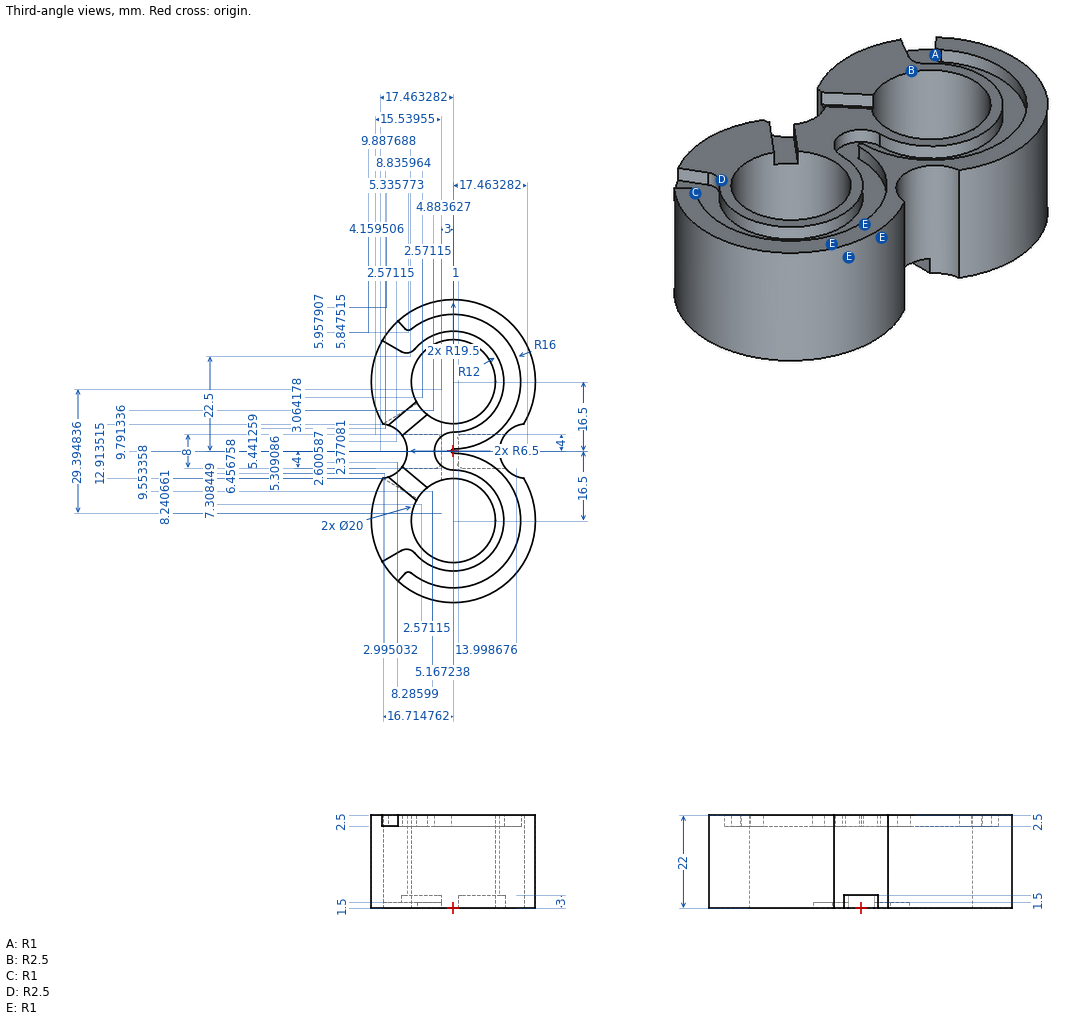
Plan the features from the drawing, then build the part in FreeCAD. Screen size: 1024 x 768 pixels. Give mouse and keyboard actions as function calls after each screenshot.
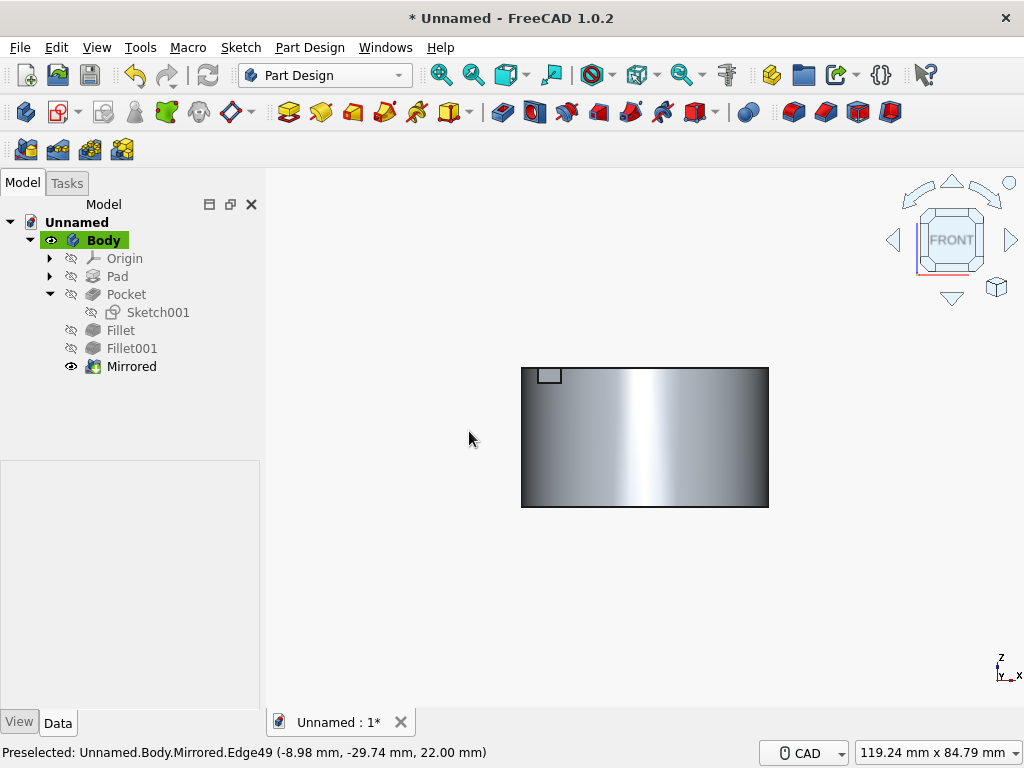
scroll(576, 375, up, 5)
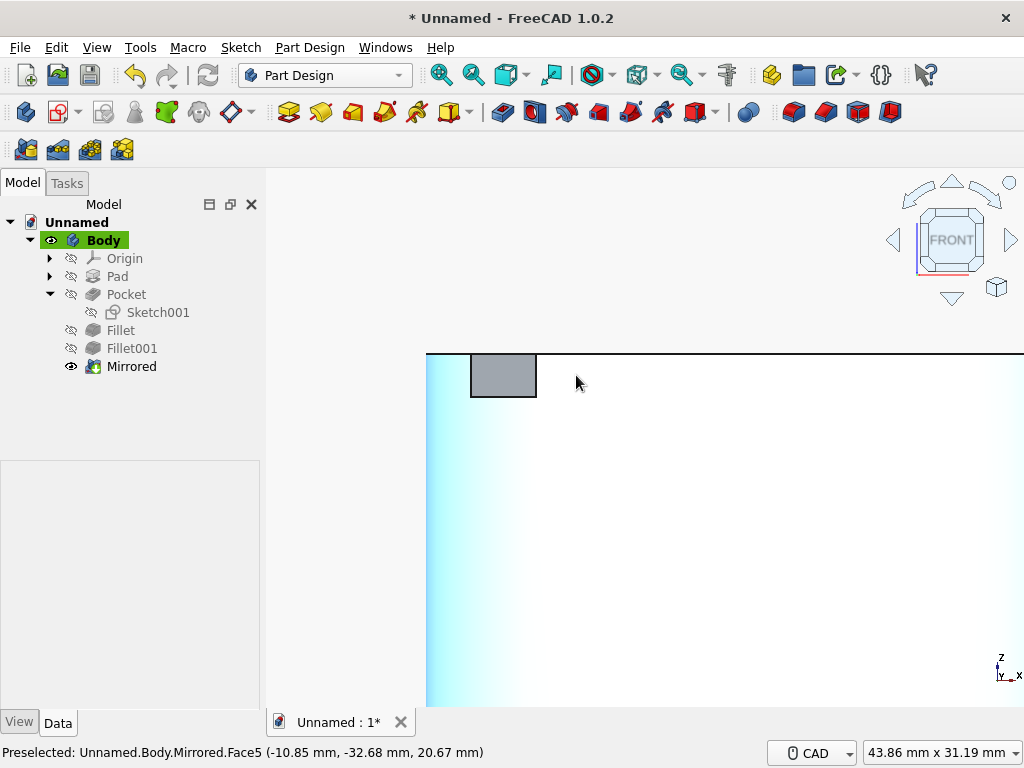
key(v)
key(f)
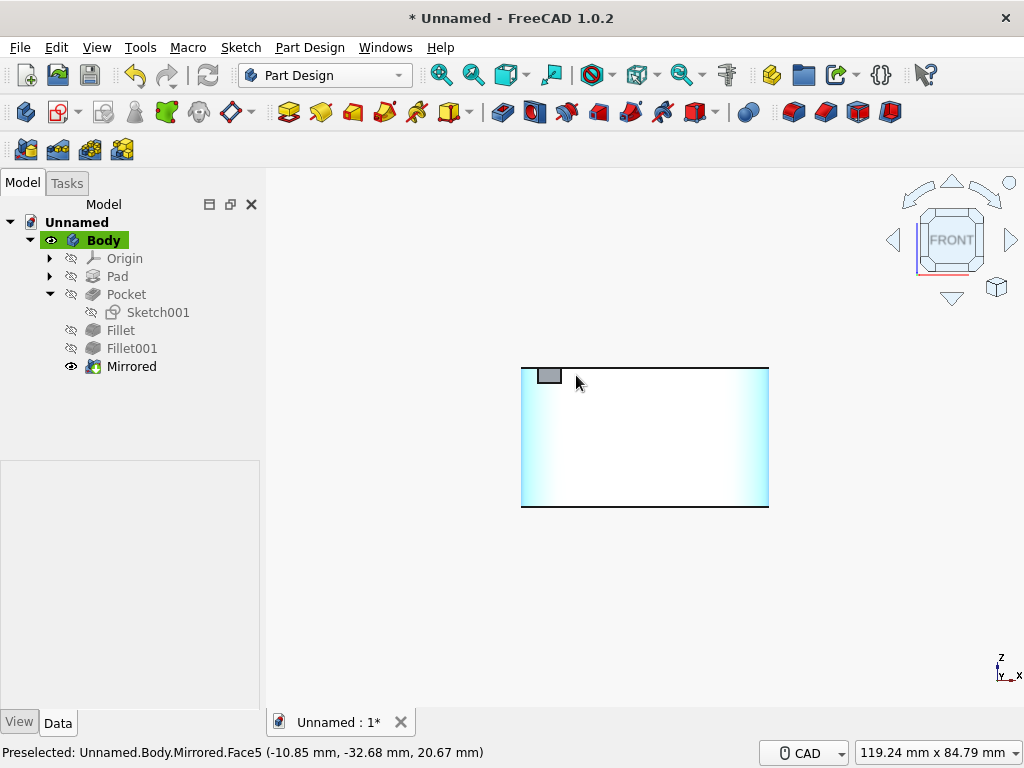
key(3)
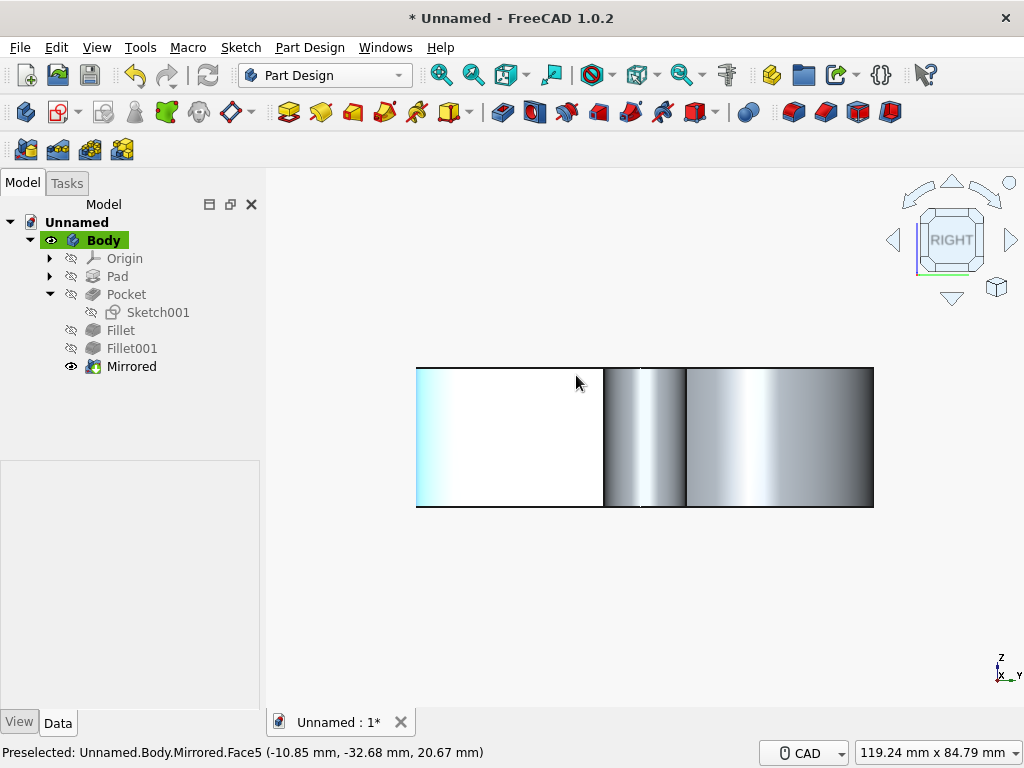
scroll(465, 375, up, 5)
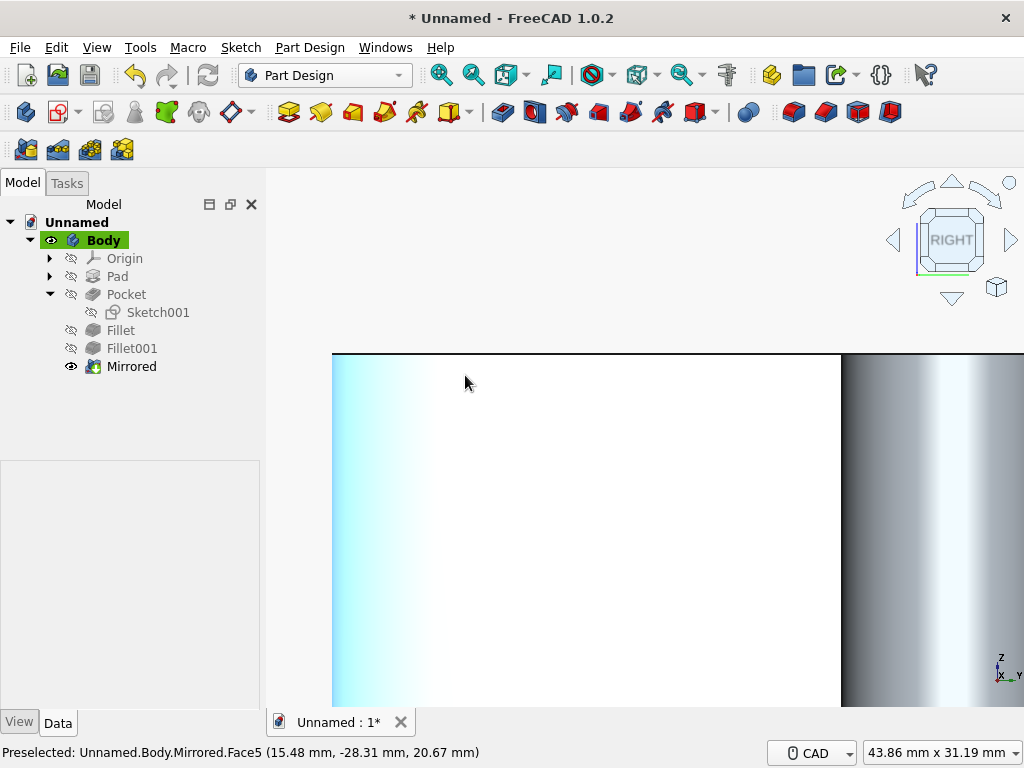
key(v)
key(f)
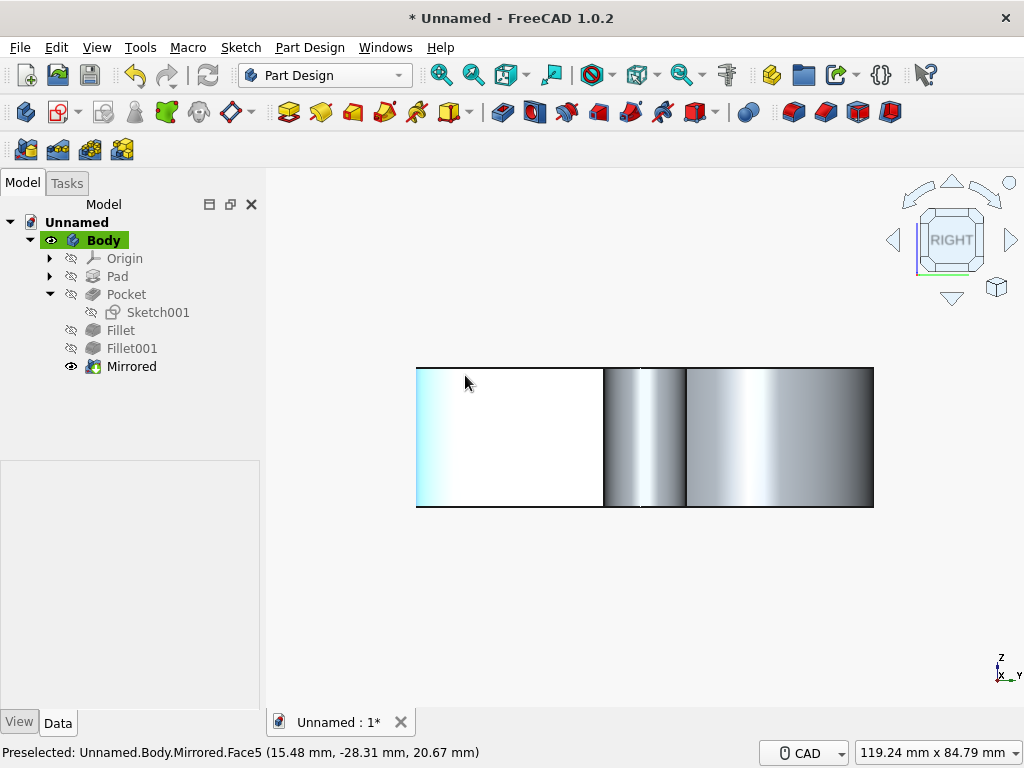
key(5)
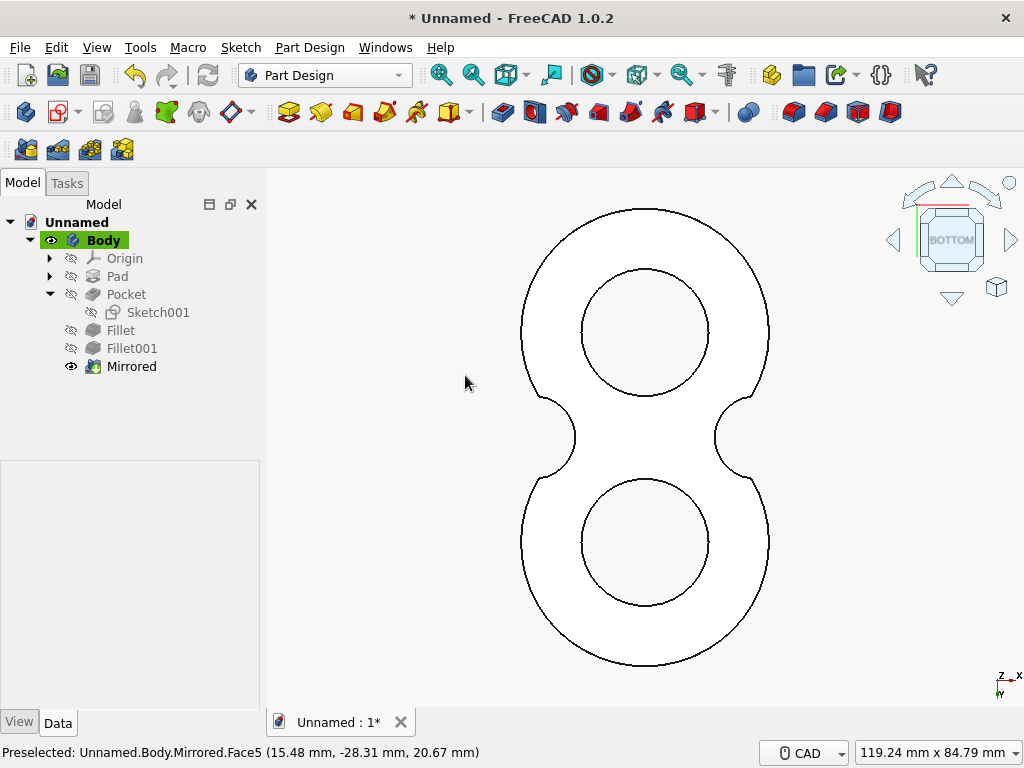
scroll(576, 256, up, 5)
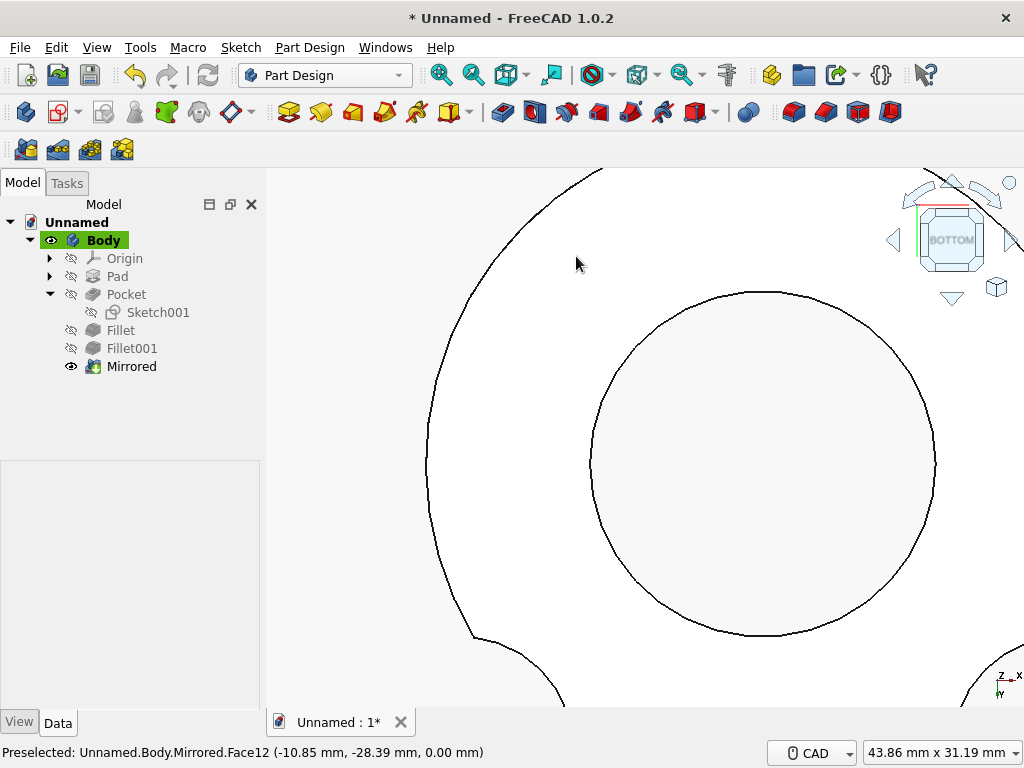
click(442, 76)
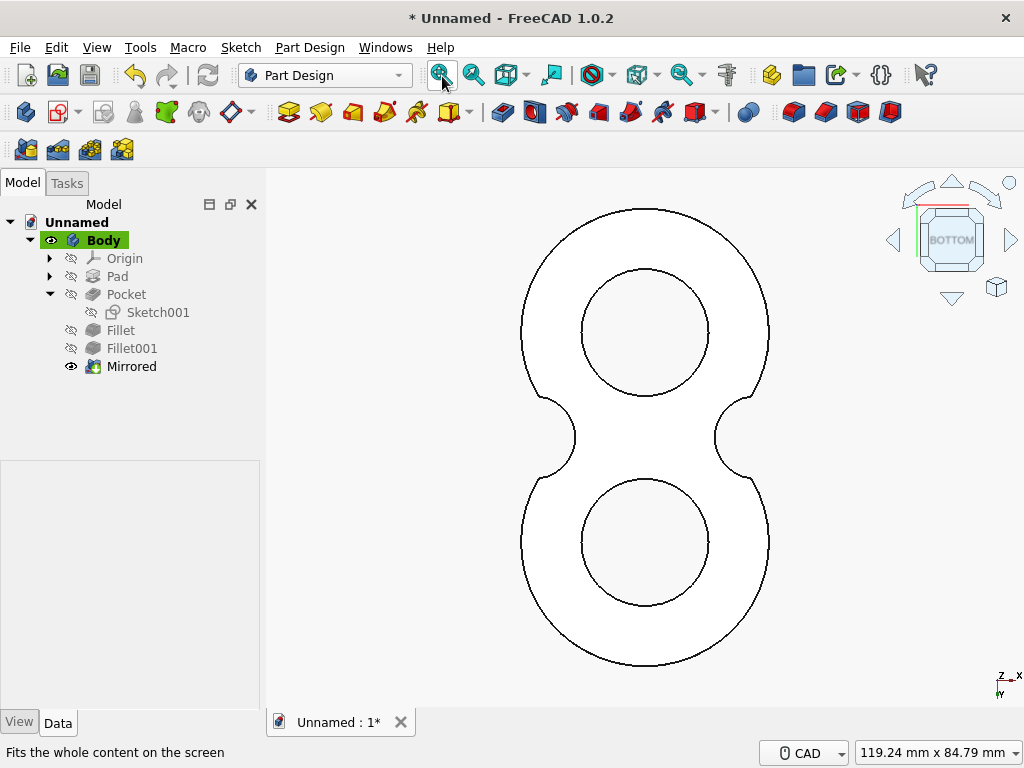
key(4)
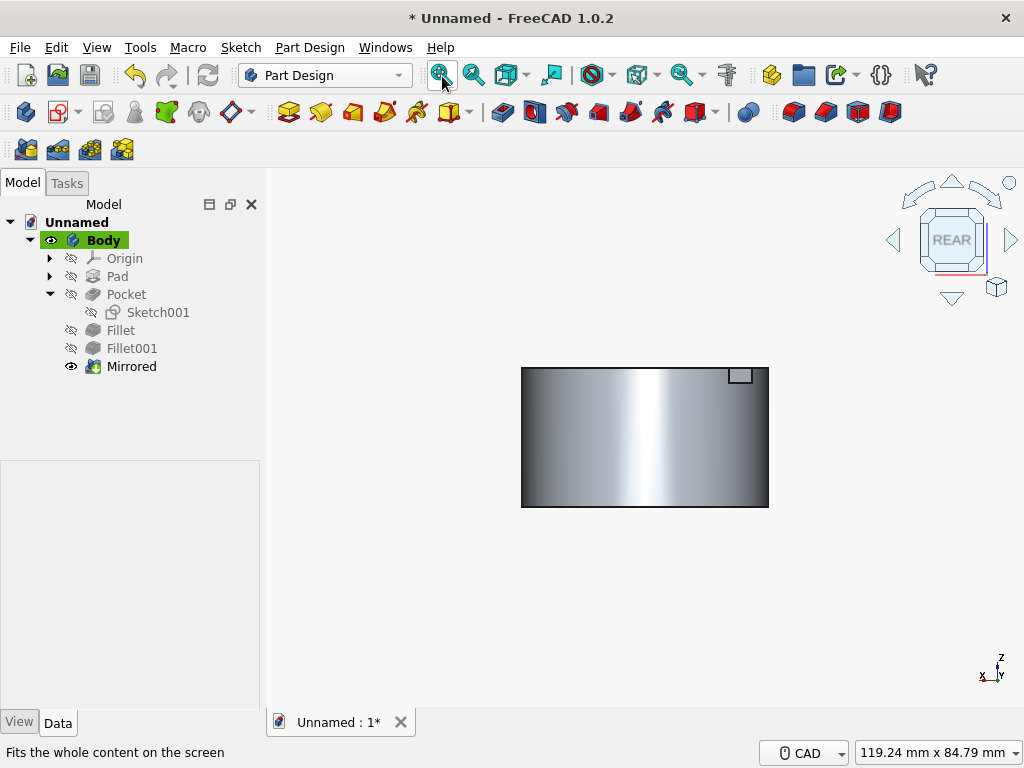
key(v)
key(f)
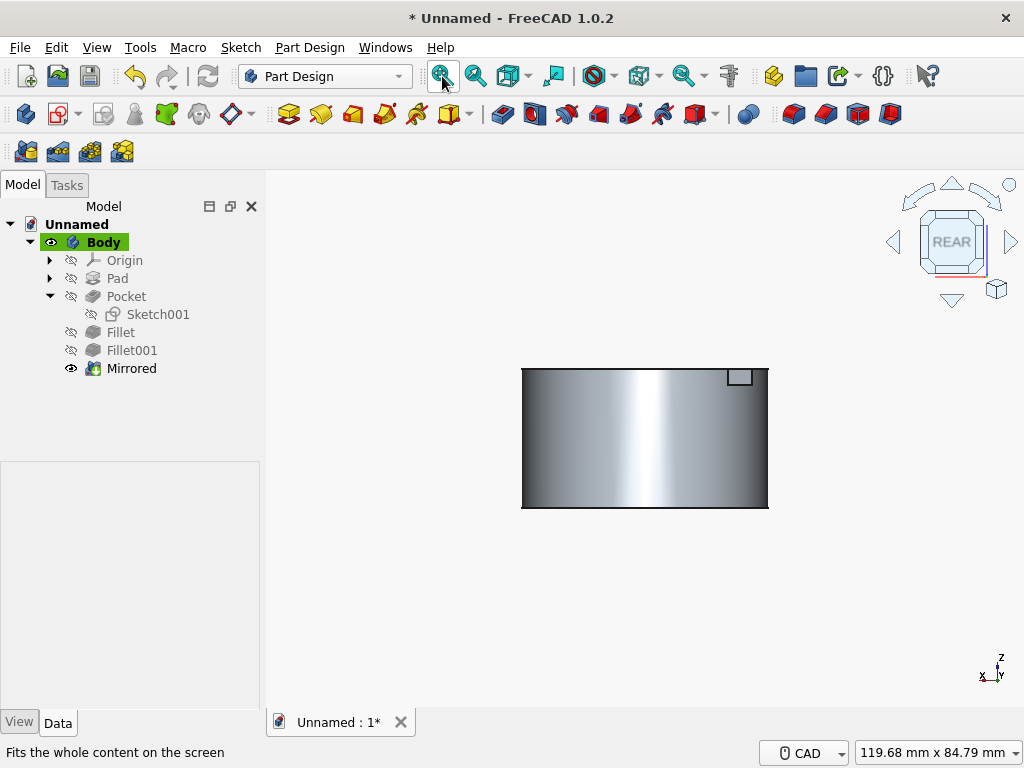
scroll(713, 376, up, 5)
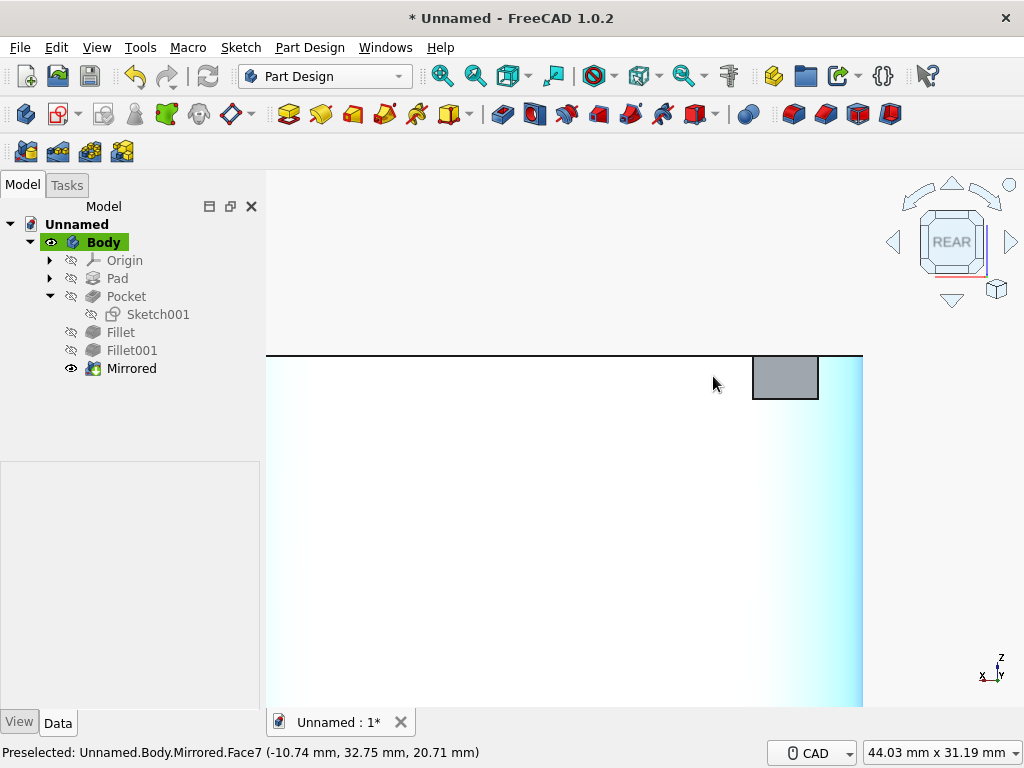
key(v)
key(f)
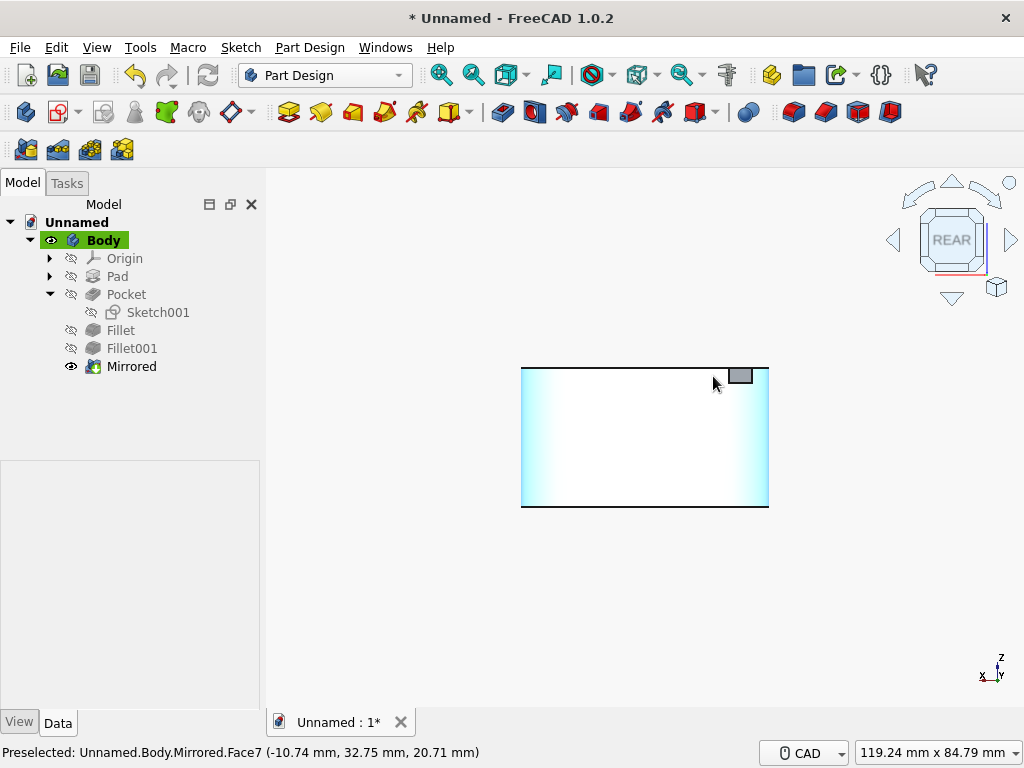
key(6)